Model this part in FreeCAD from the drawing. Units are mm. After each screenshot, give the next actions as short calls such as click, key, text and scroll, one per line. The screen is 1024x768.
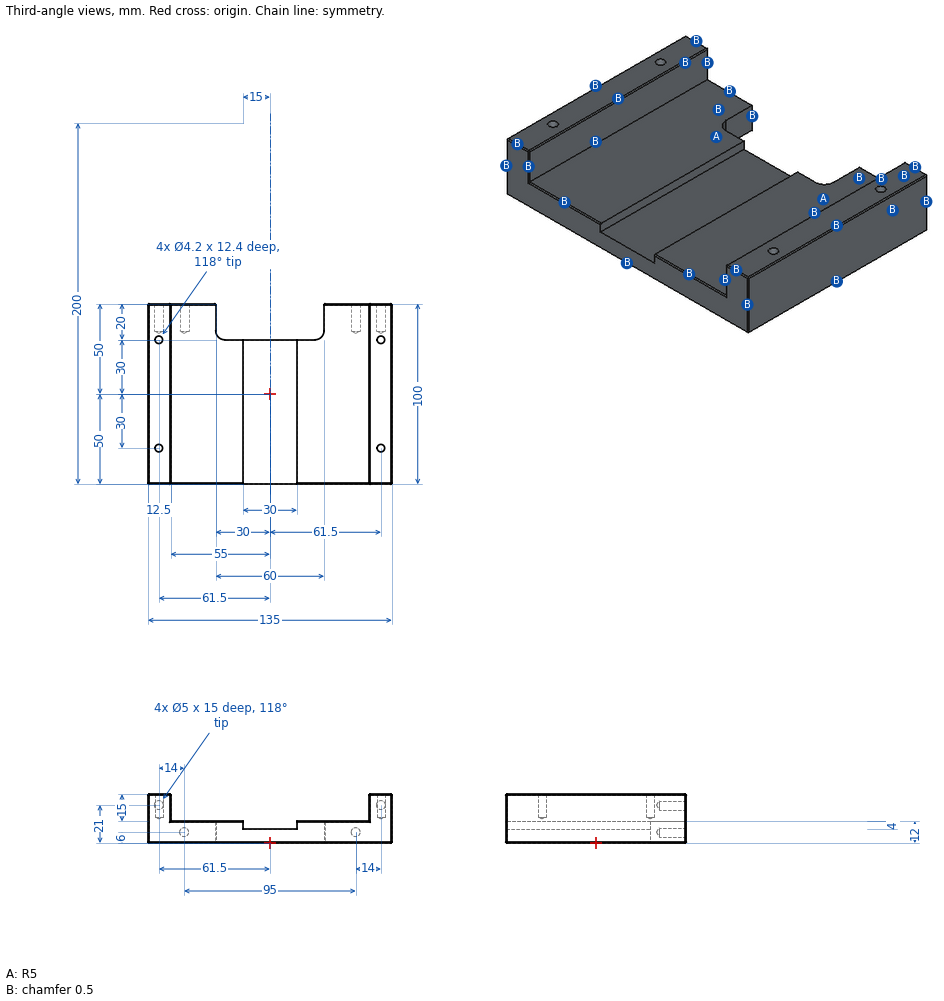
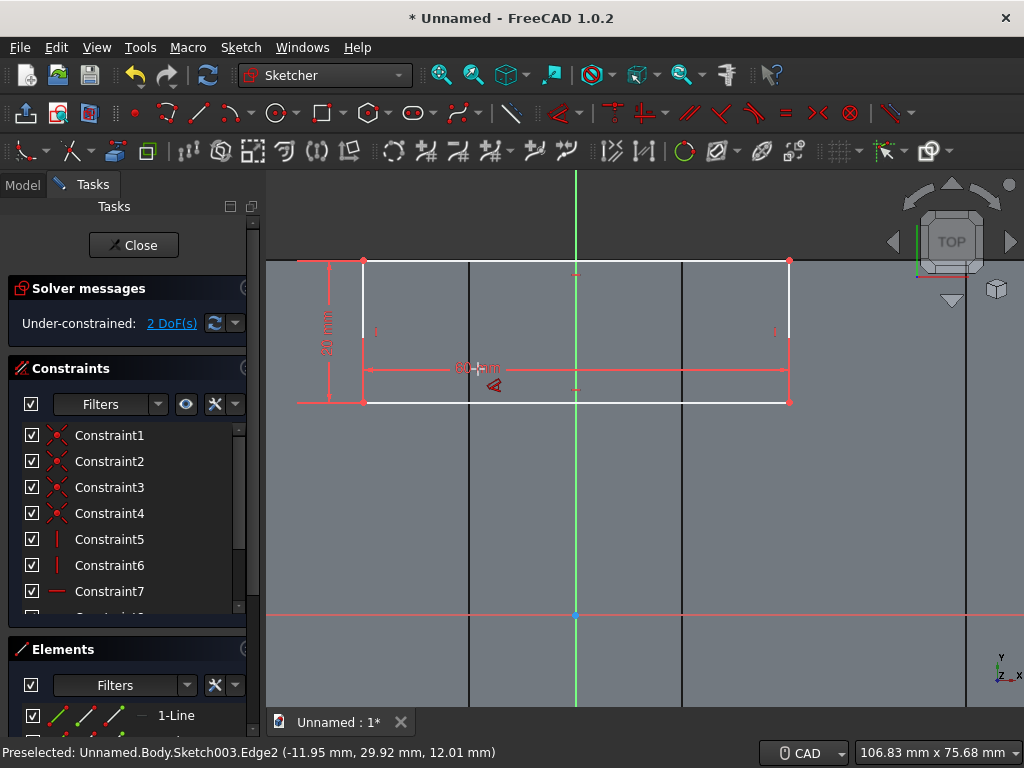
click(363, 261)
click(470, 649)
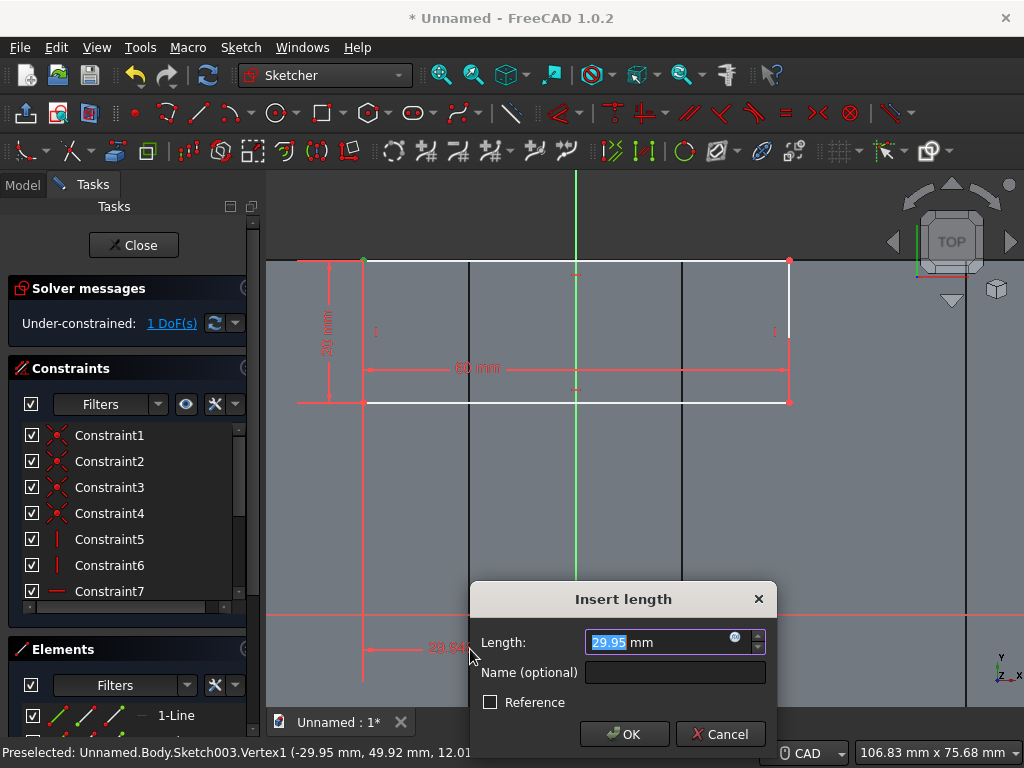
text(30)
key(Return)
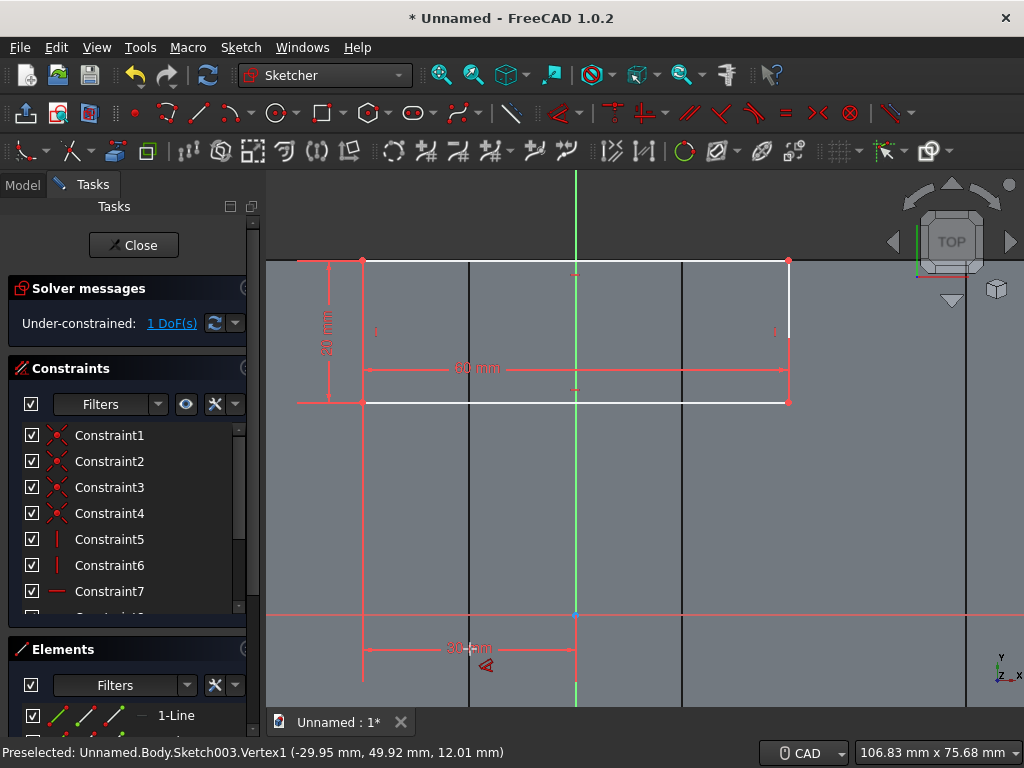
click(363, 261)
click(329, 438)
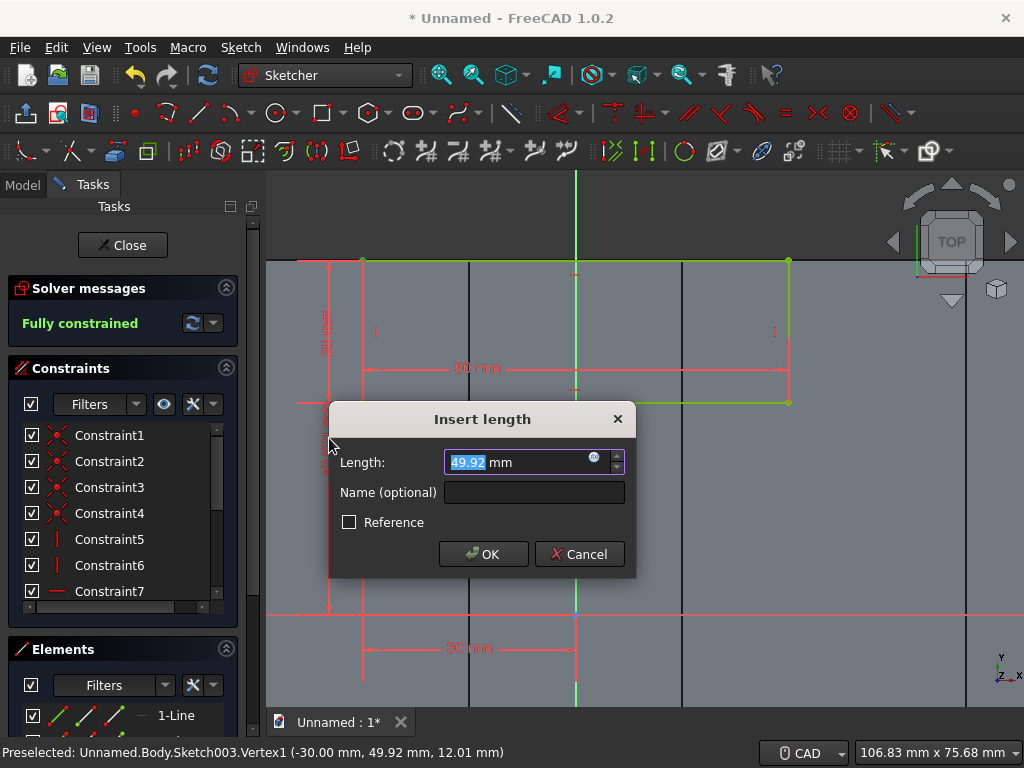
text(50)
key(Return)
key(Escape)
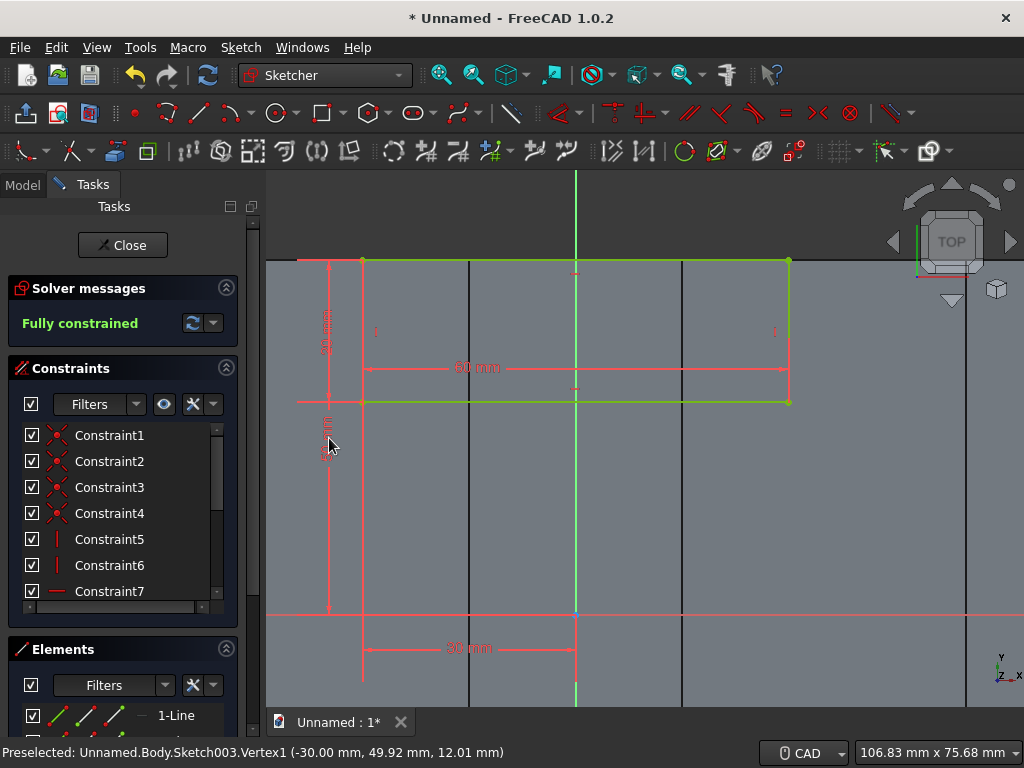
click(123, 245)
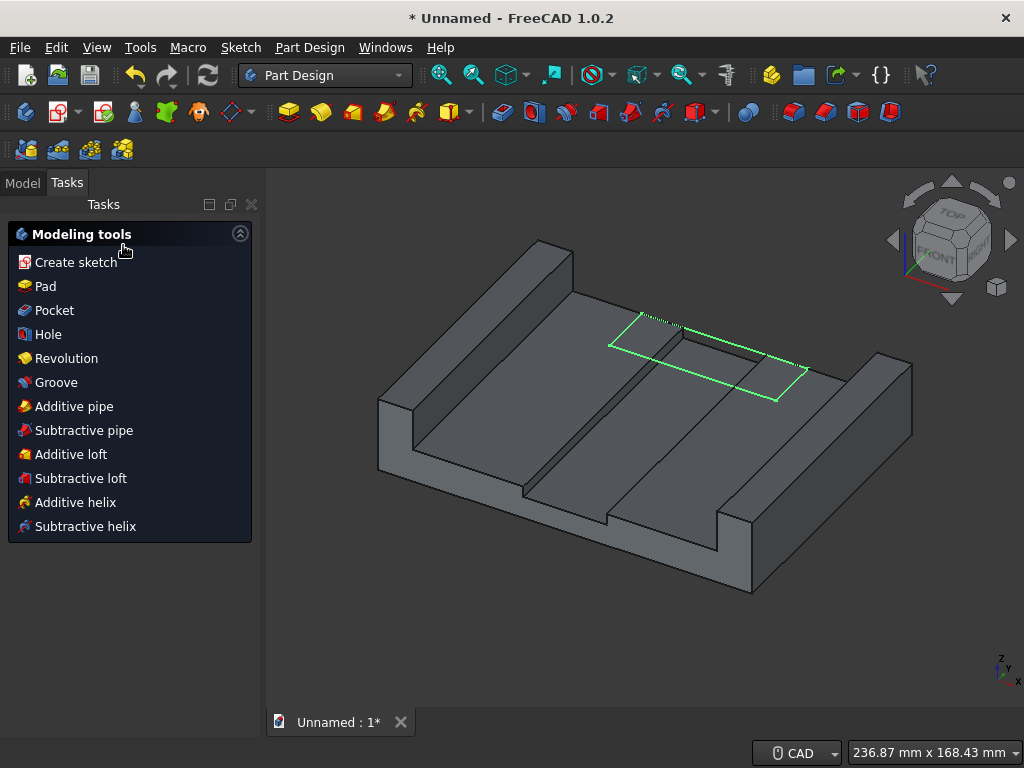
click(504, 112)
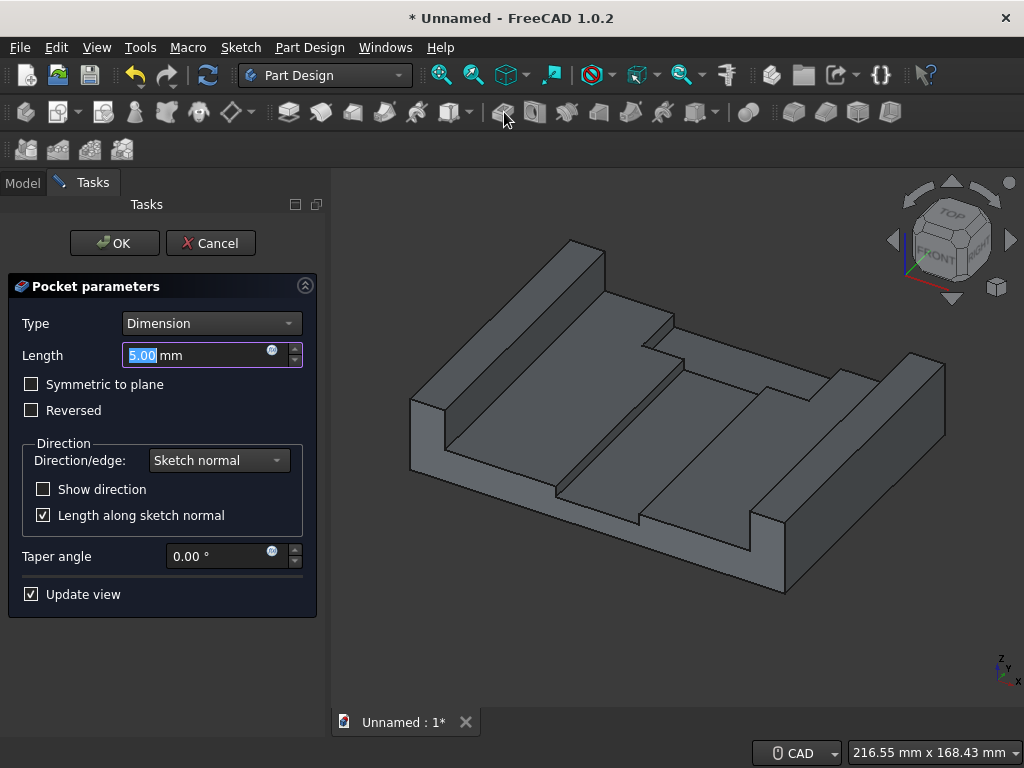
click(212, 324)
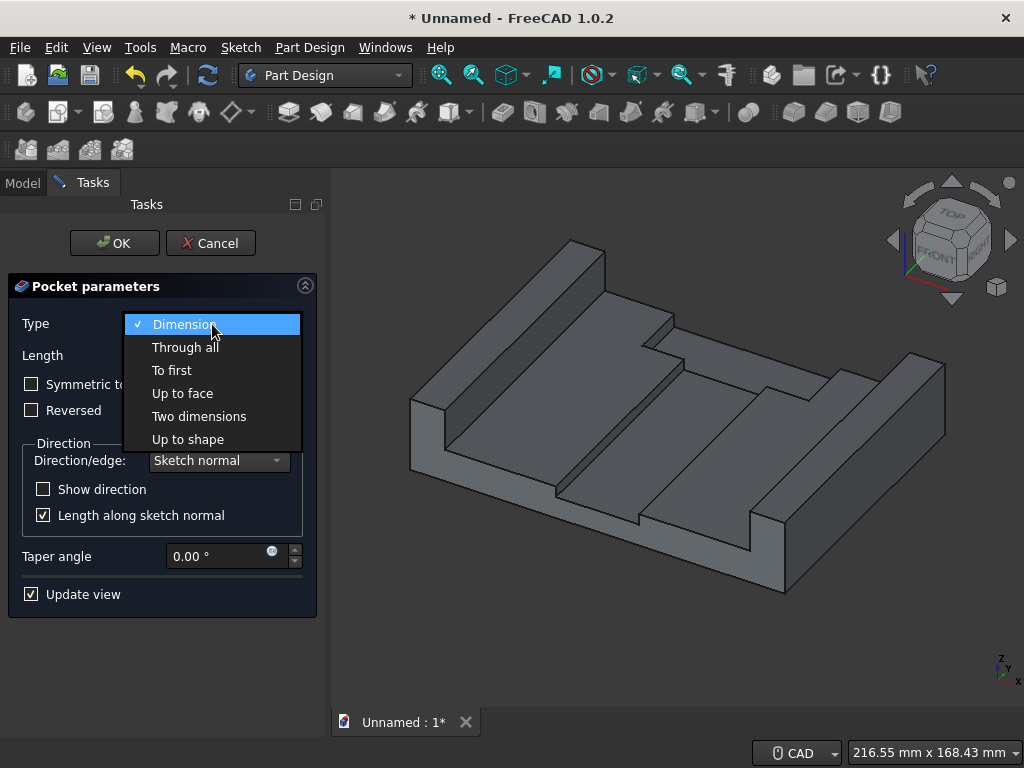
click(212, 348)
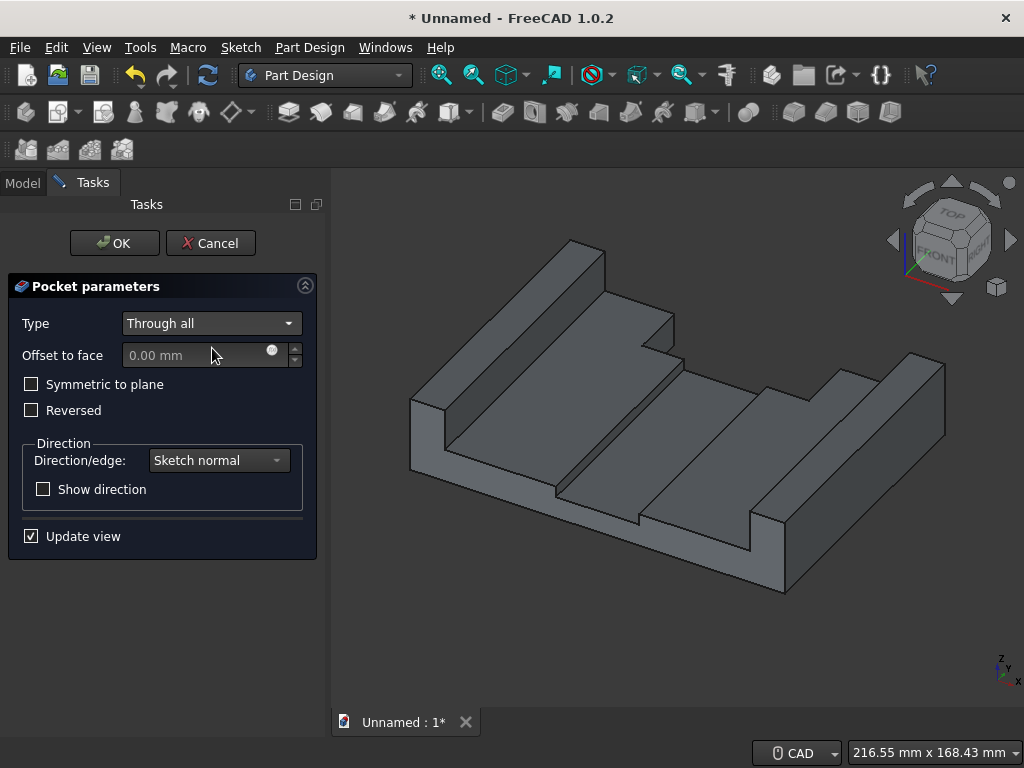
click(115, 243)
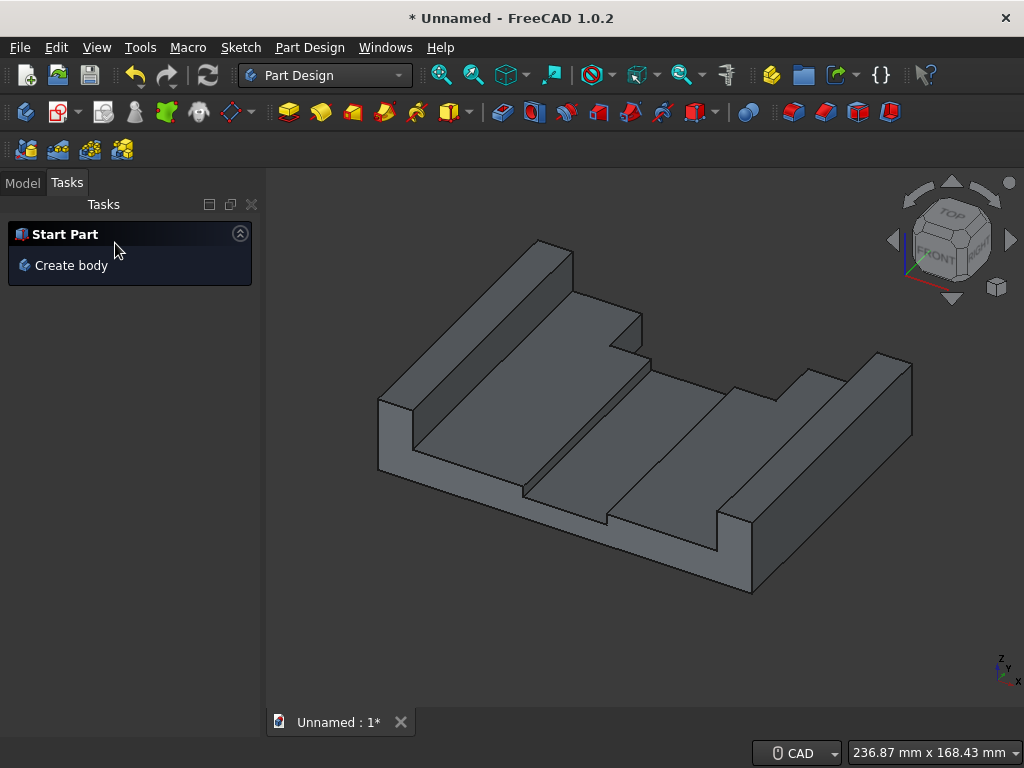
key(0)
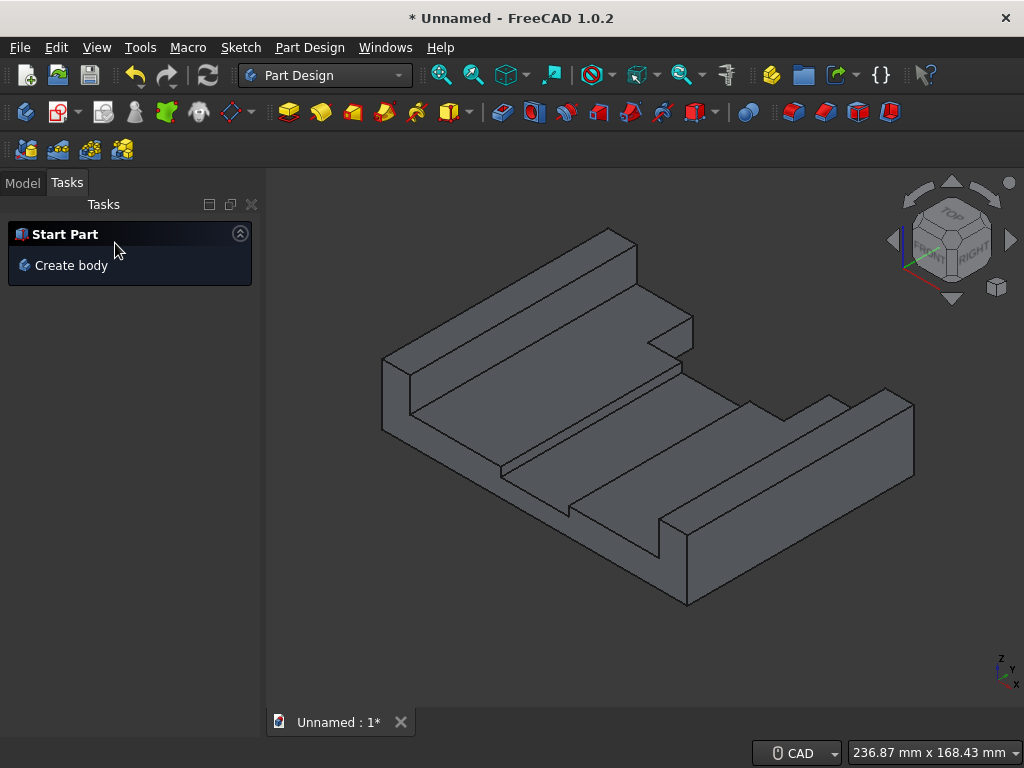
key(2)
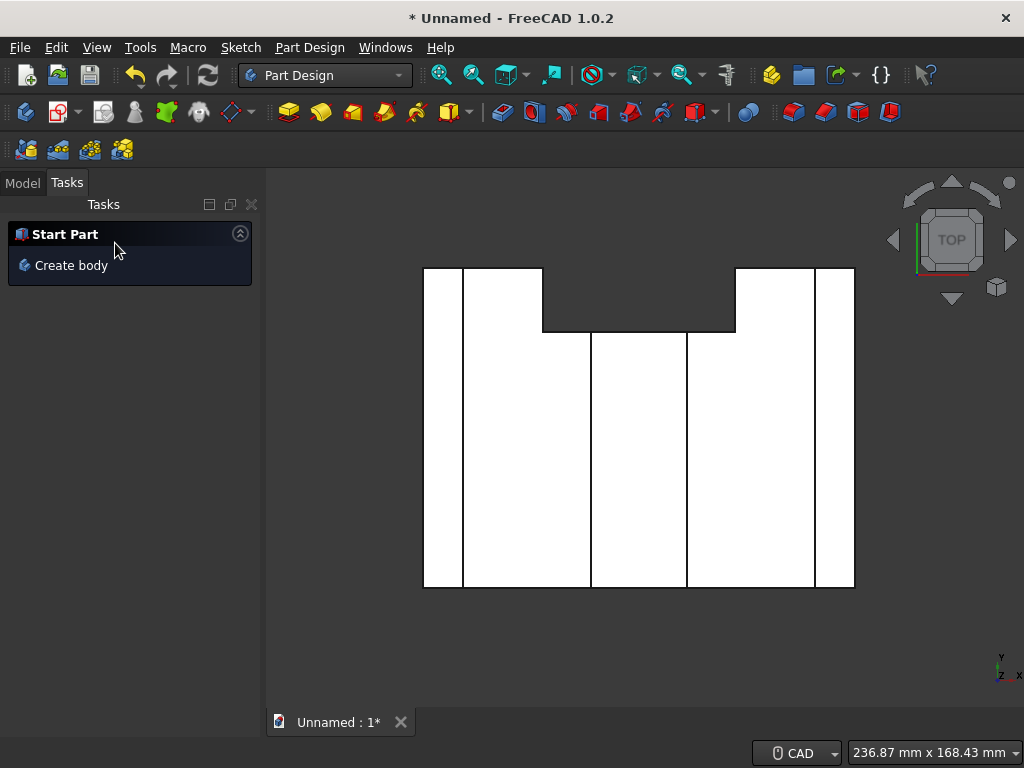
key(1)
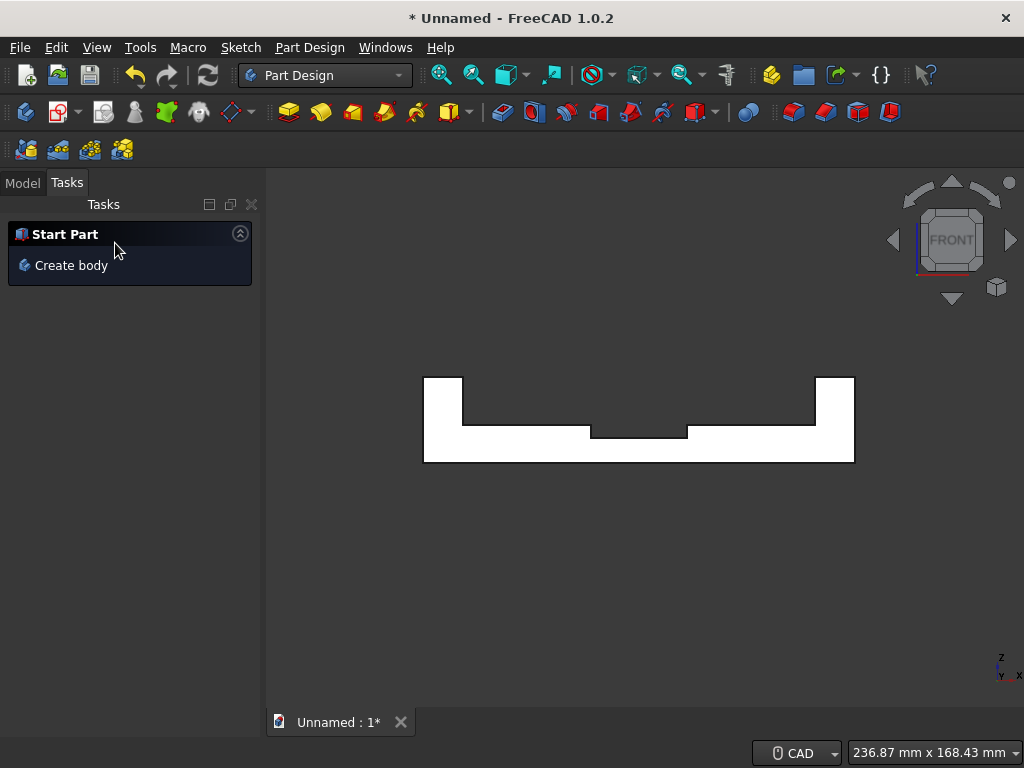
key(3)